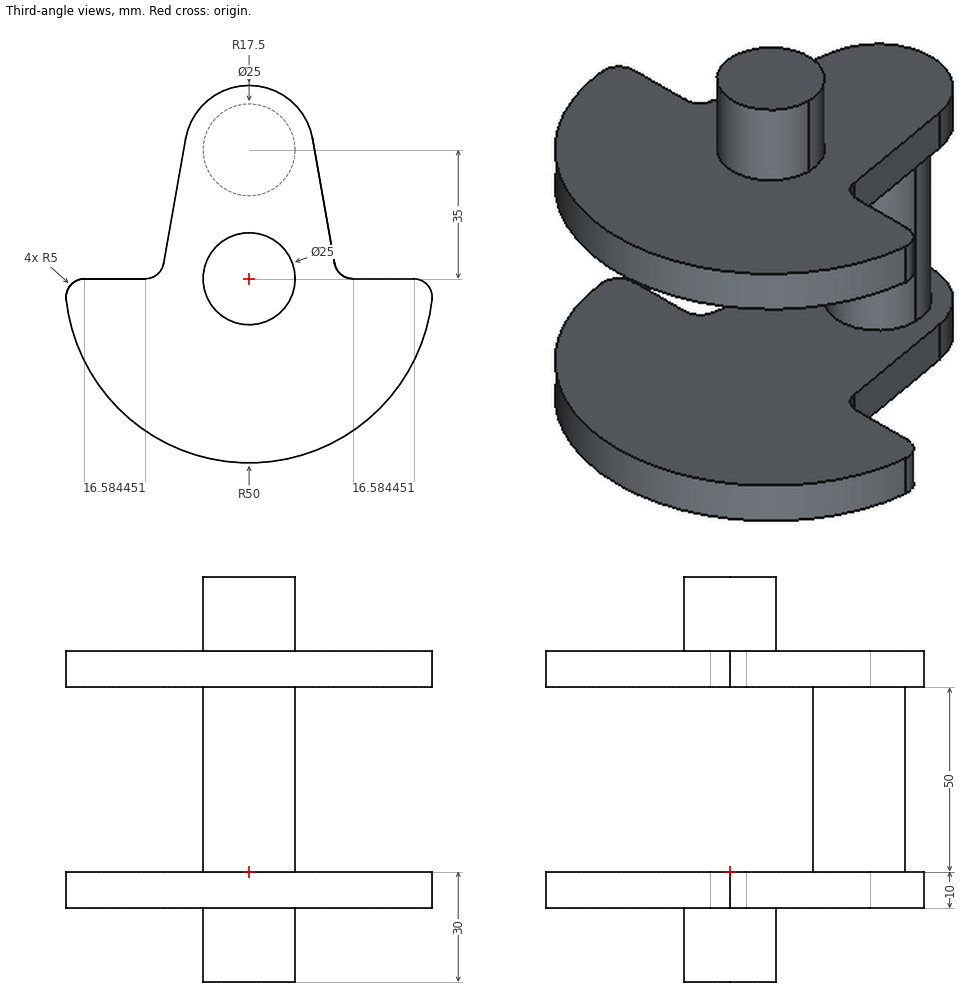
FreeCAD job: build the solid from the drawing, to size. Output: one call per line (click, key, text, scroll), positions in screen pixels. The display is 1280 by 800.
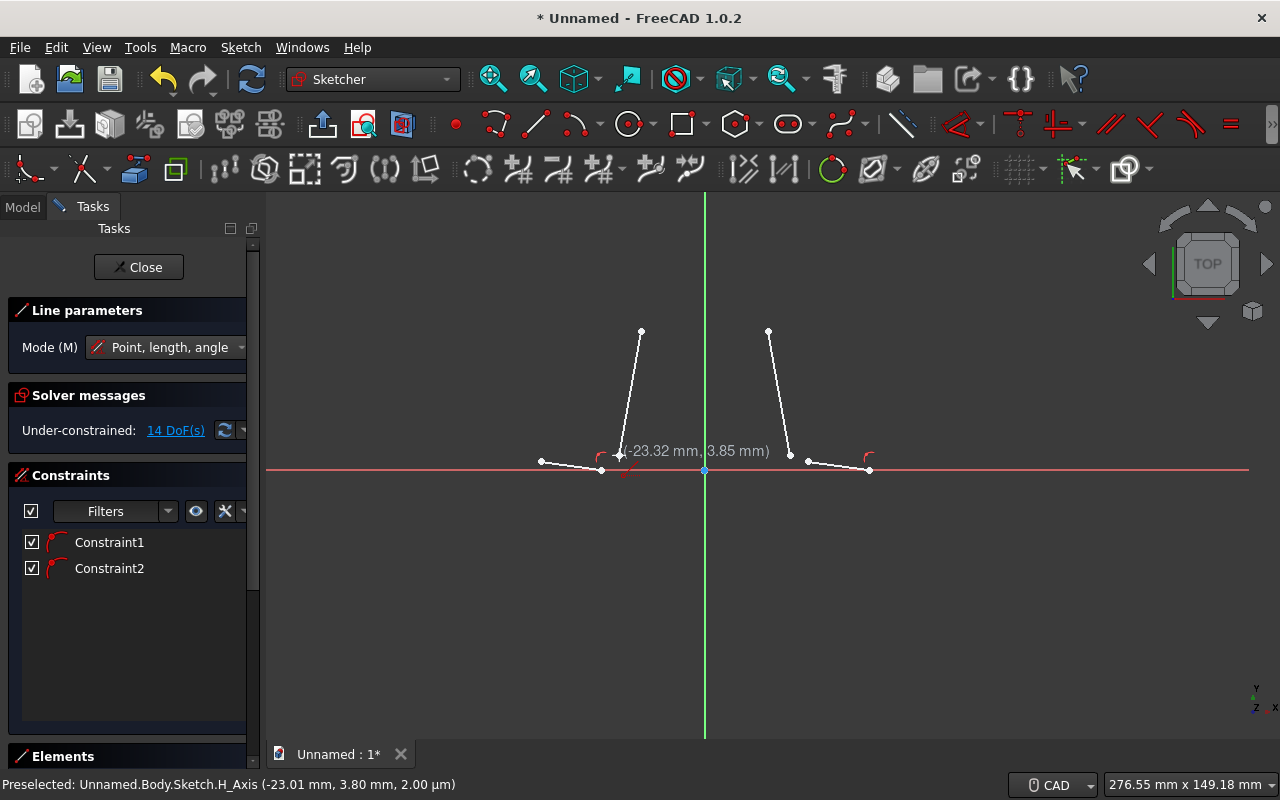
key(g)
key(3)
key(a)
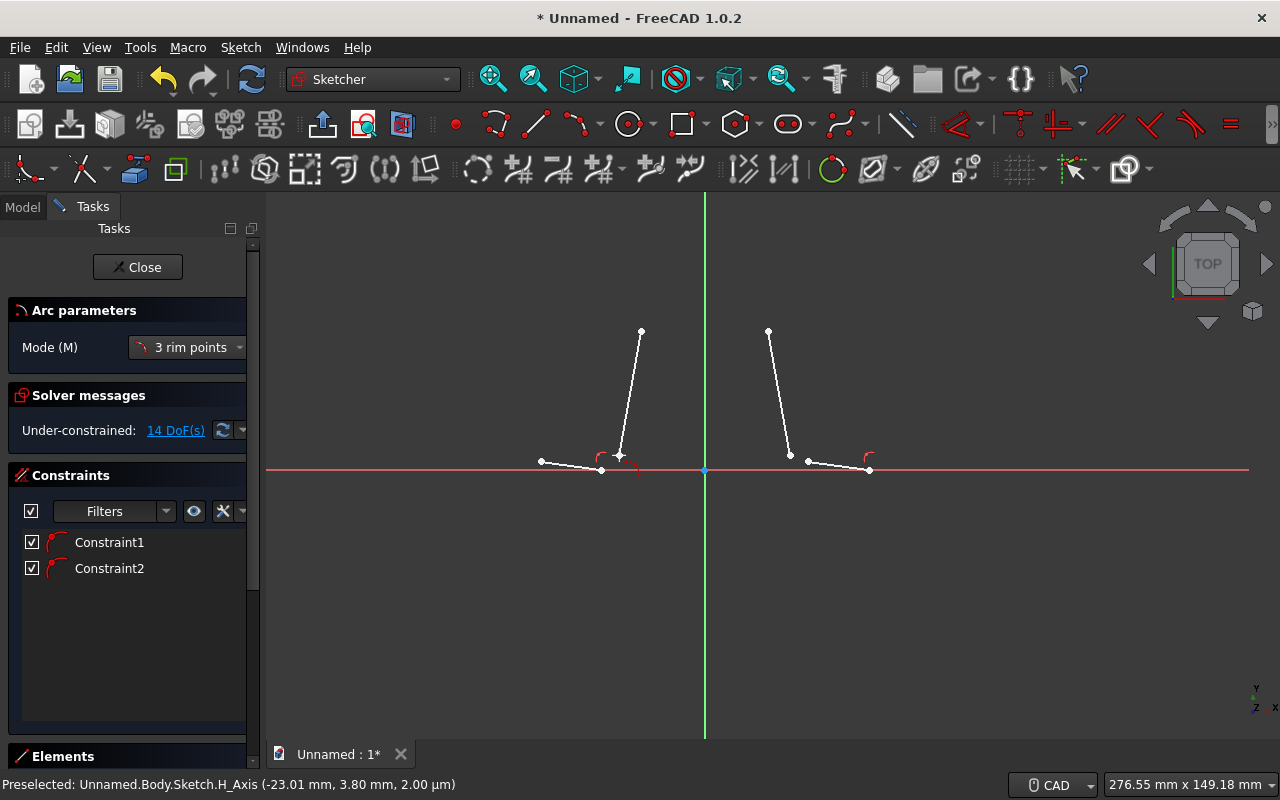
click(541, 462)
click(522, 490)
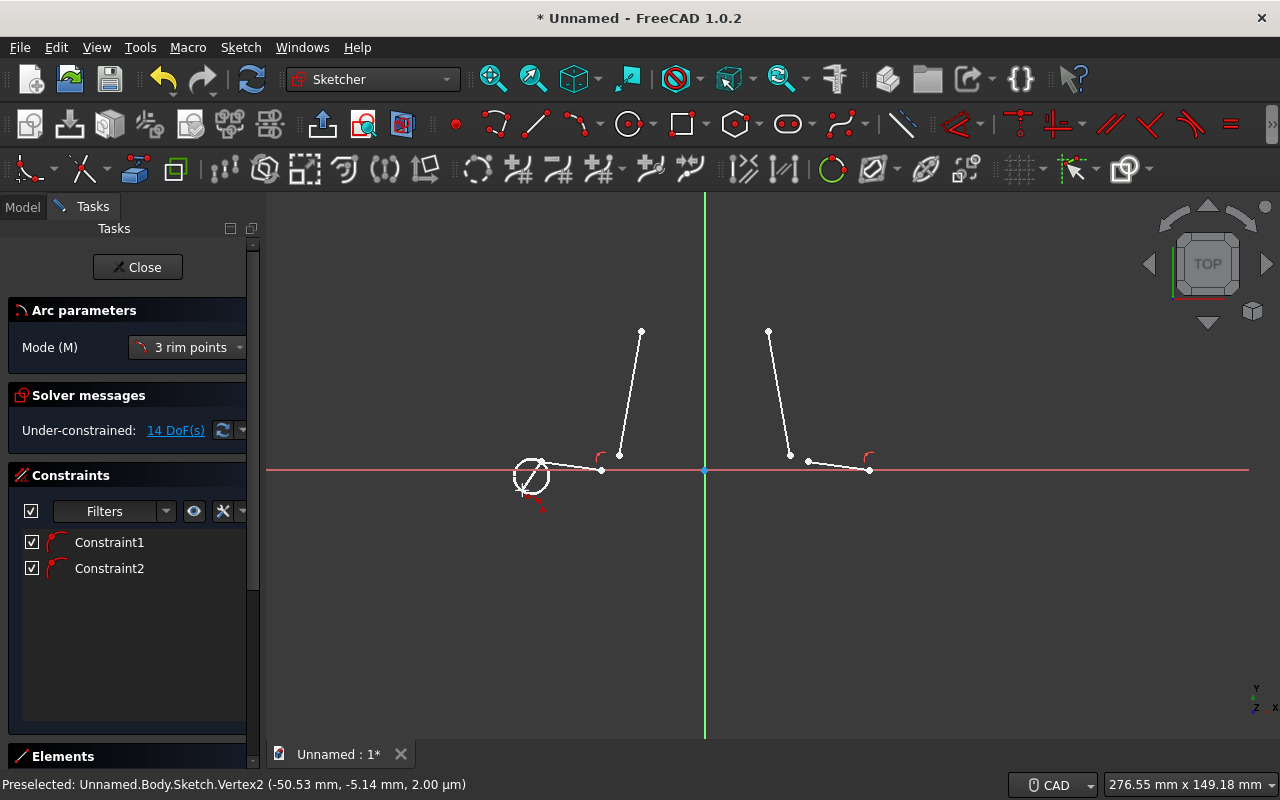
scroll(527, 476, up, 5)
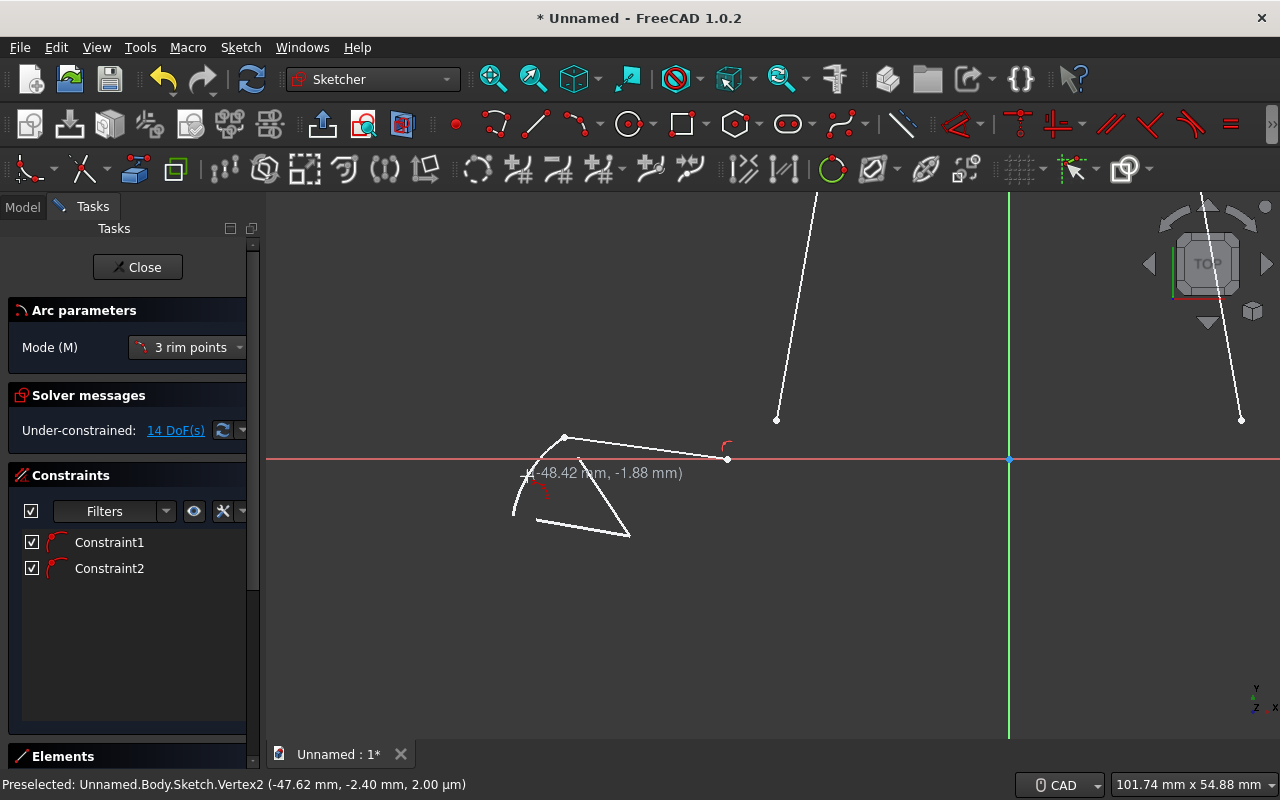
click(526, 476)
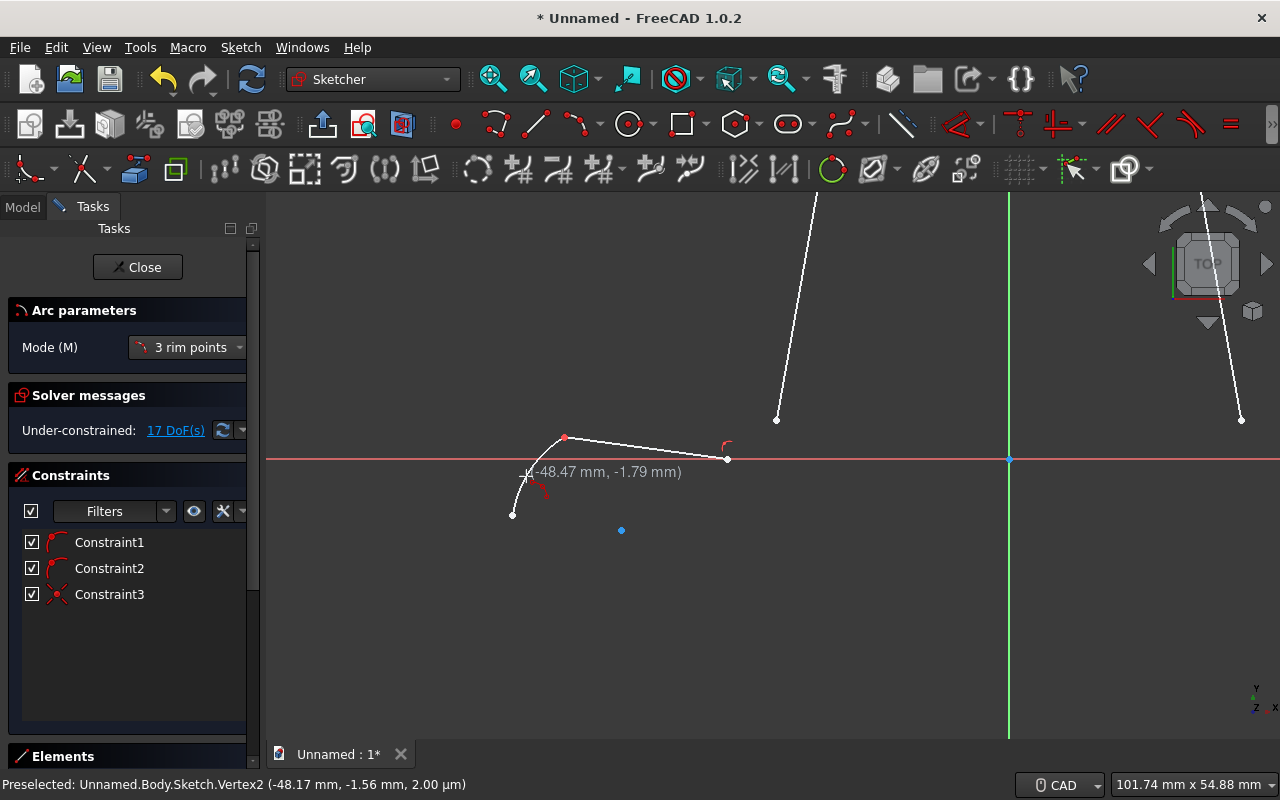
click(513, 516)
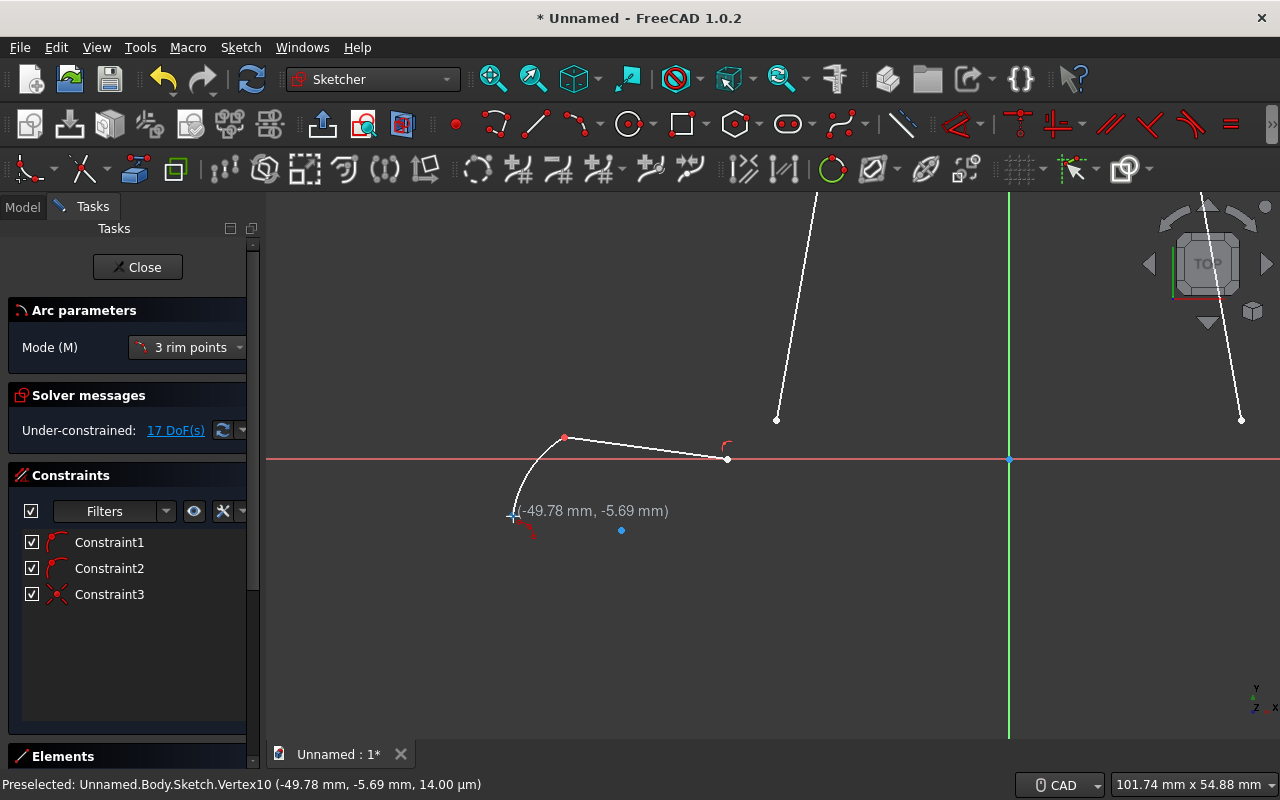
scroll(527, 476, down, 5)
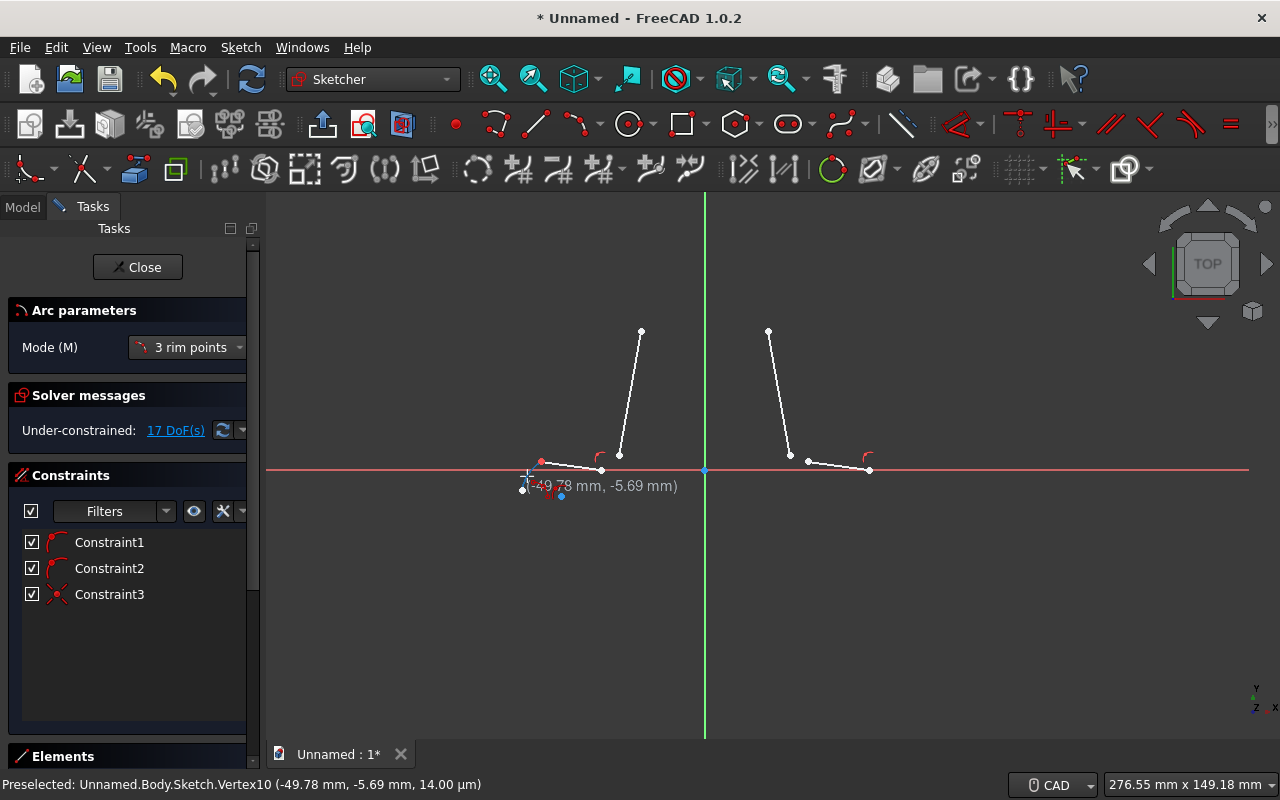
click(887, 490)
click(652, 646)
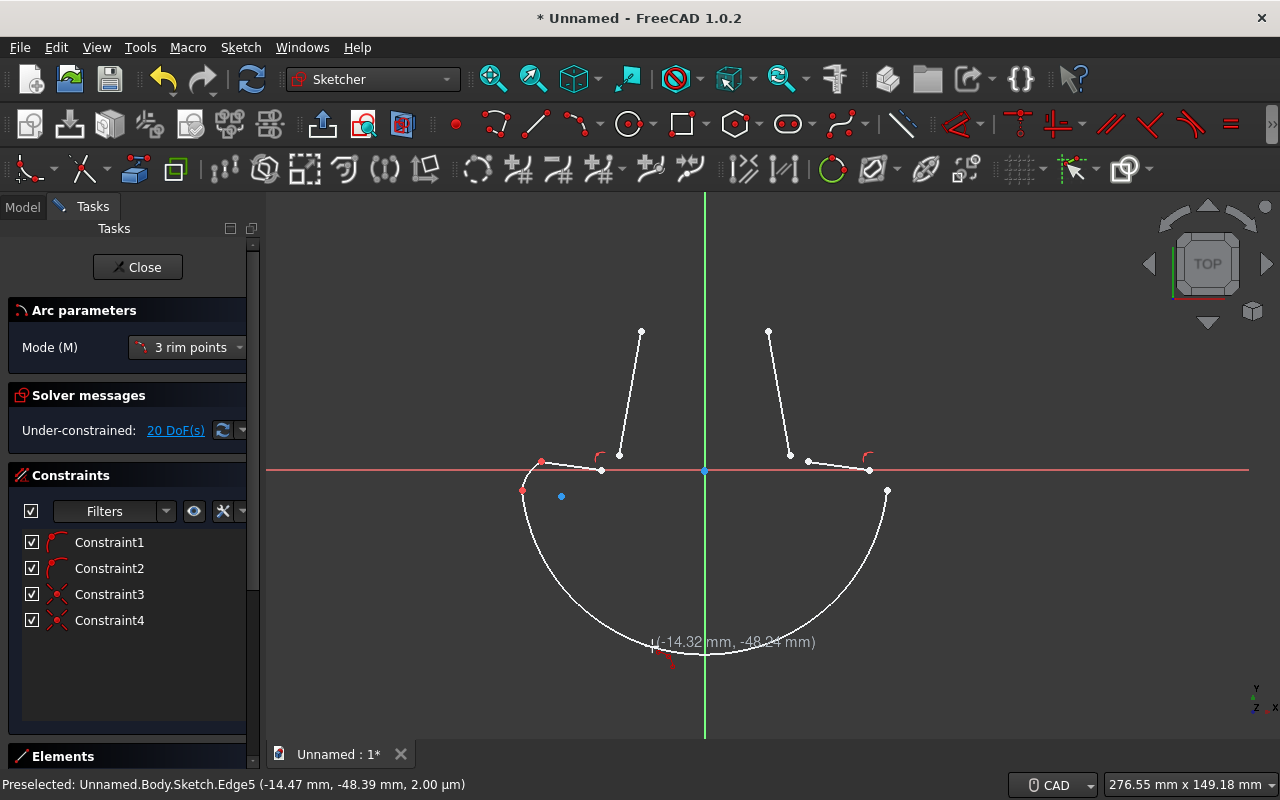
click(887, 491)
click(869, 470)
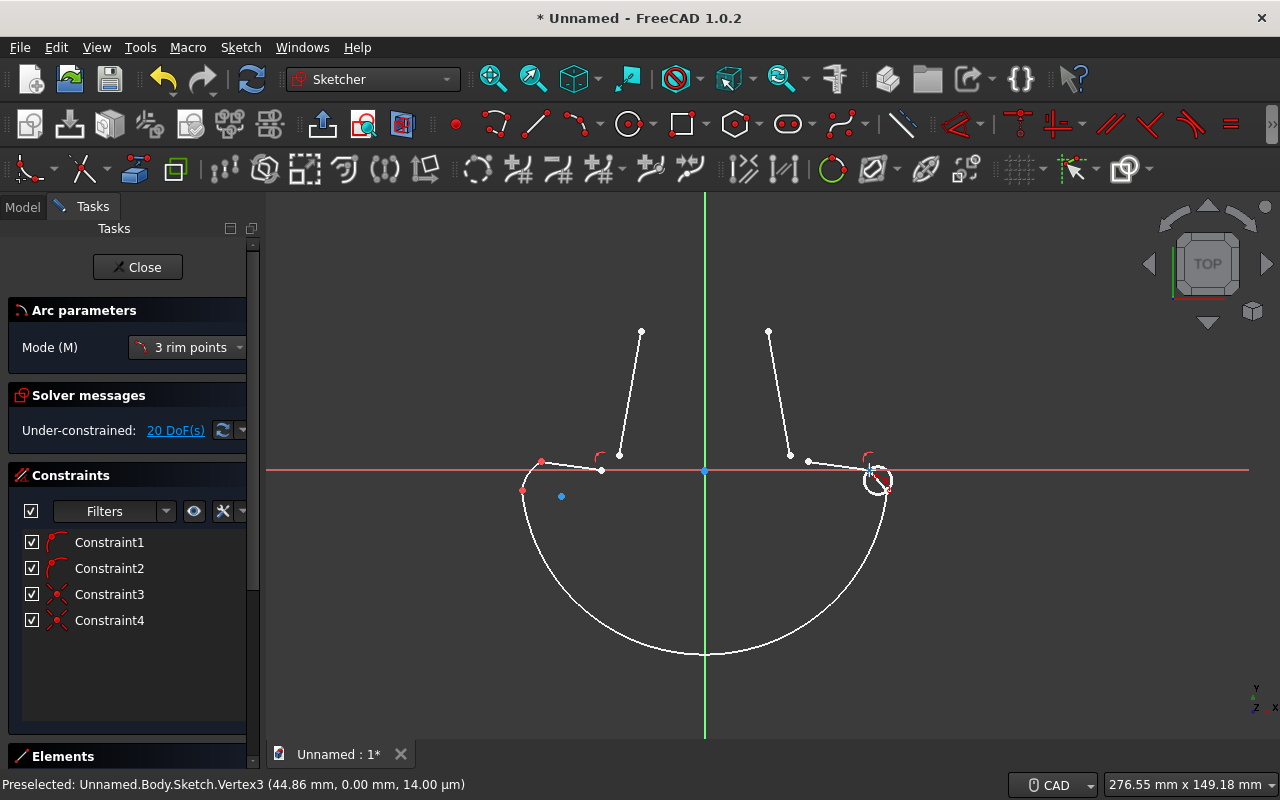
scroll(882, 476, up, 5)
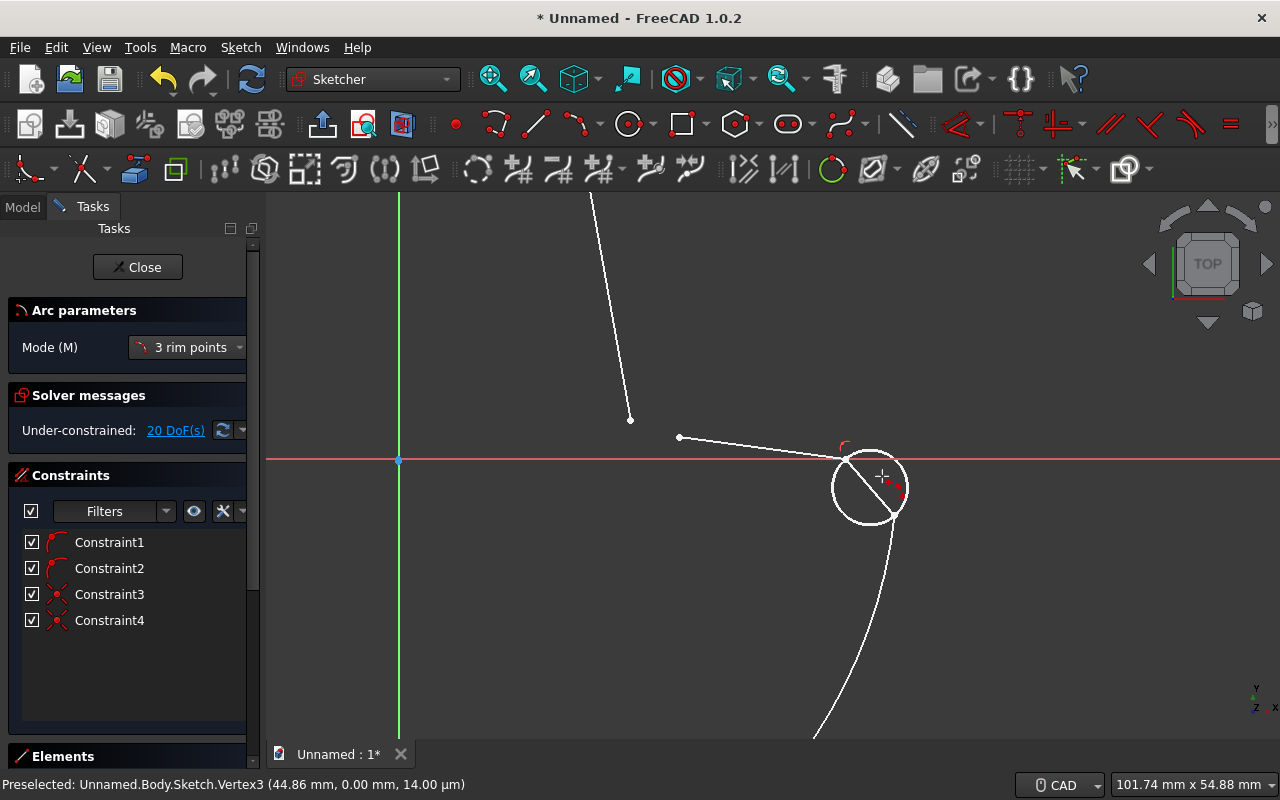
click(881, 476)